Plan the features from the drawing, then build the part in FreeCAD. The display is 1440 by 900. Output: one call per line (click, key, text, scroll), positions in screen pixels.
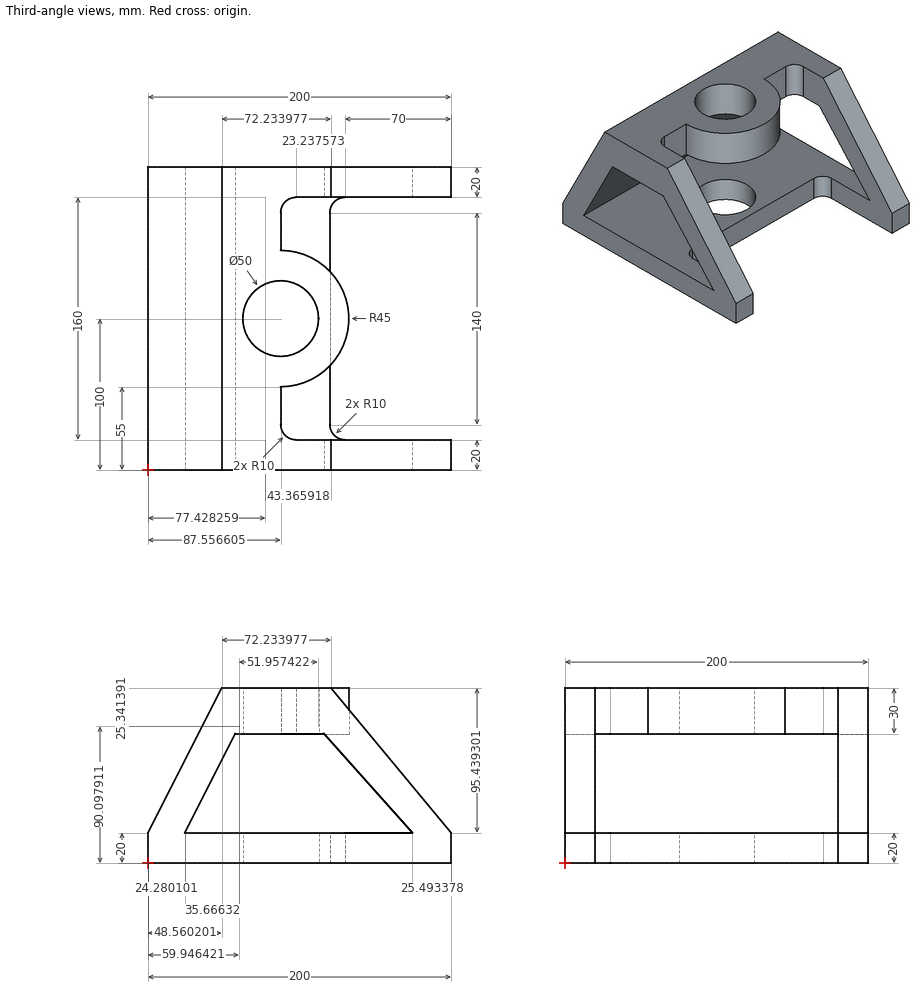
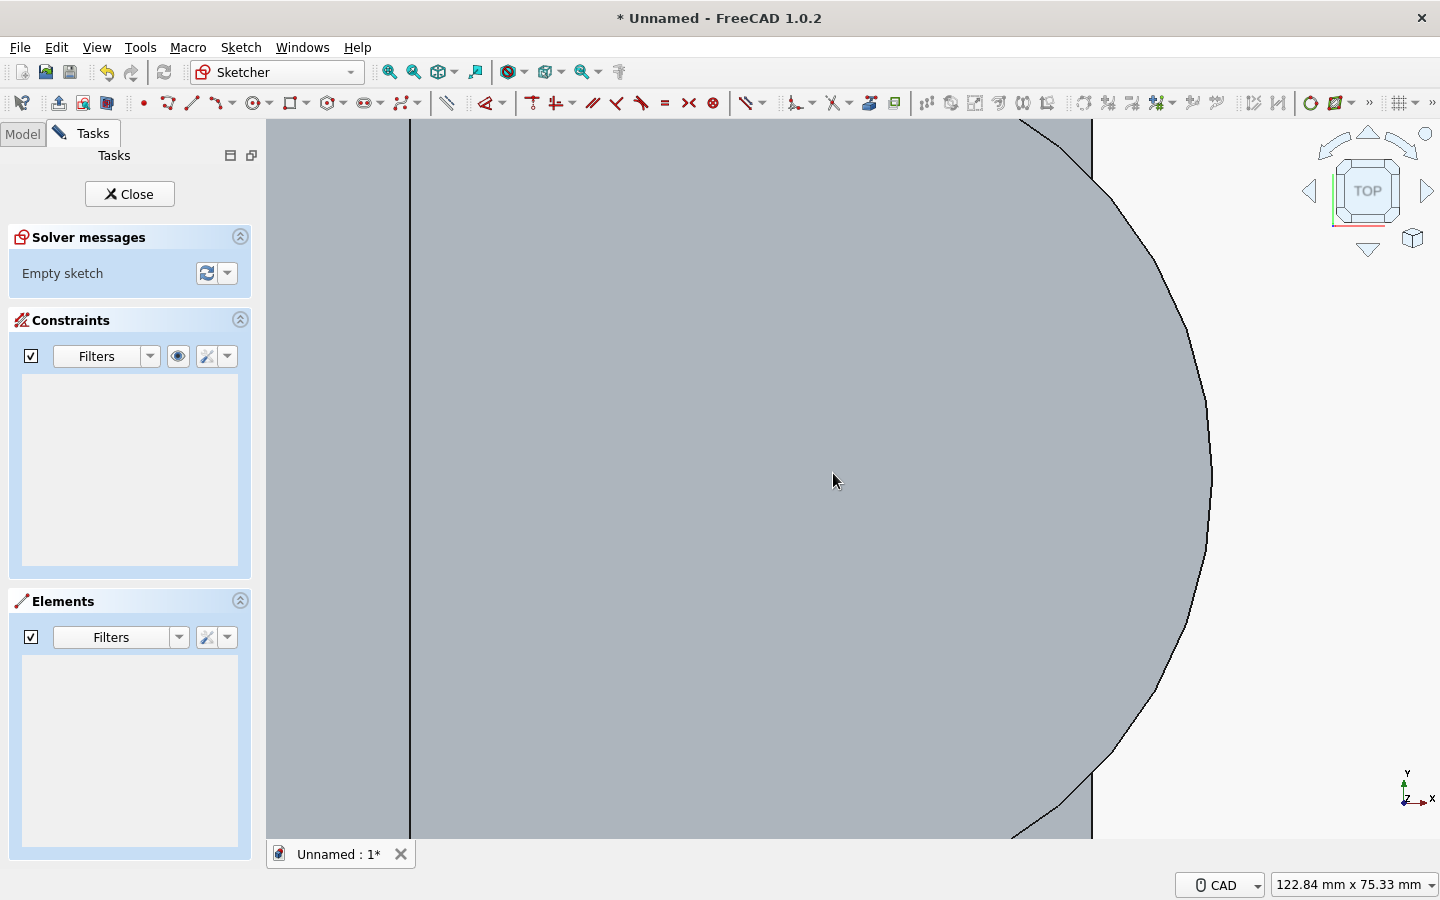
click(254, 104)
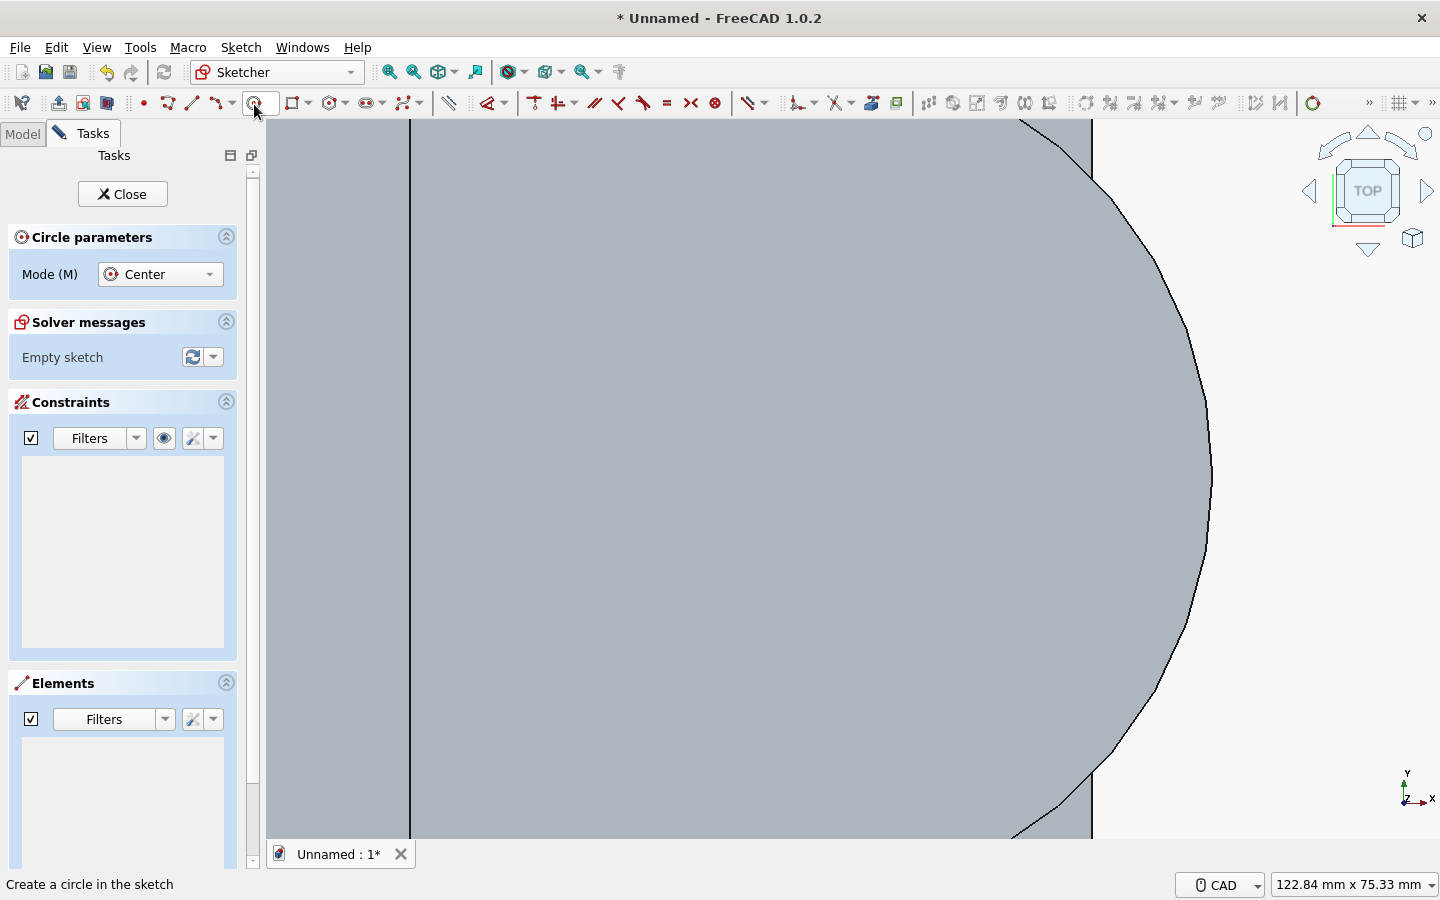
click(782, 476)
click(951, 307)
key(Escape)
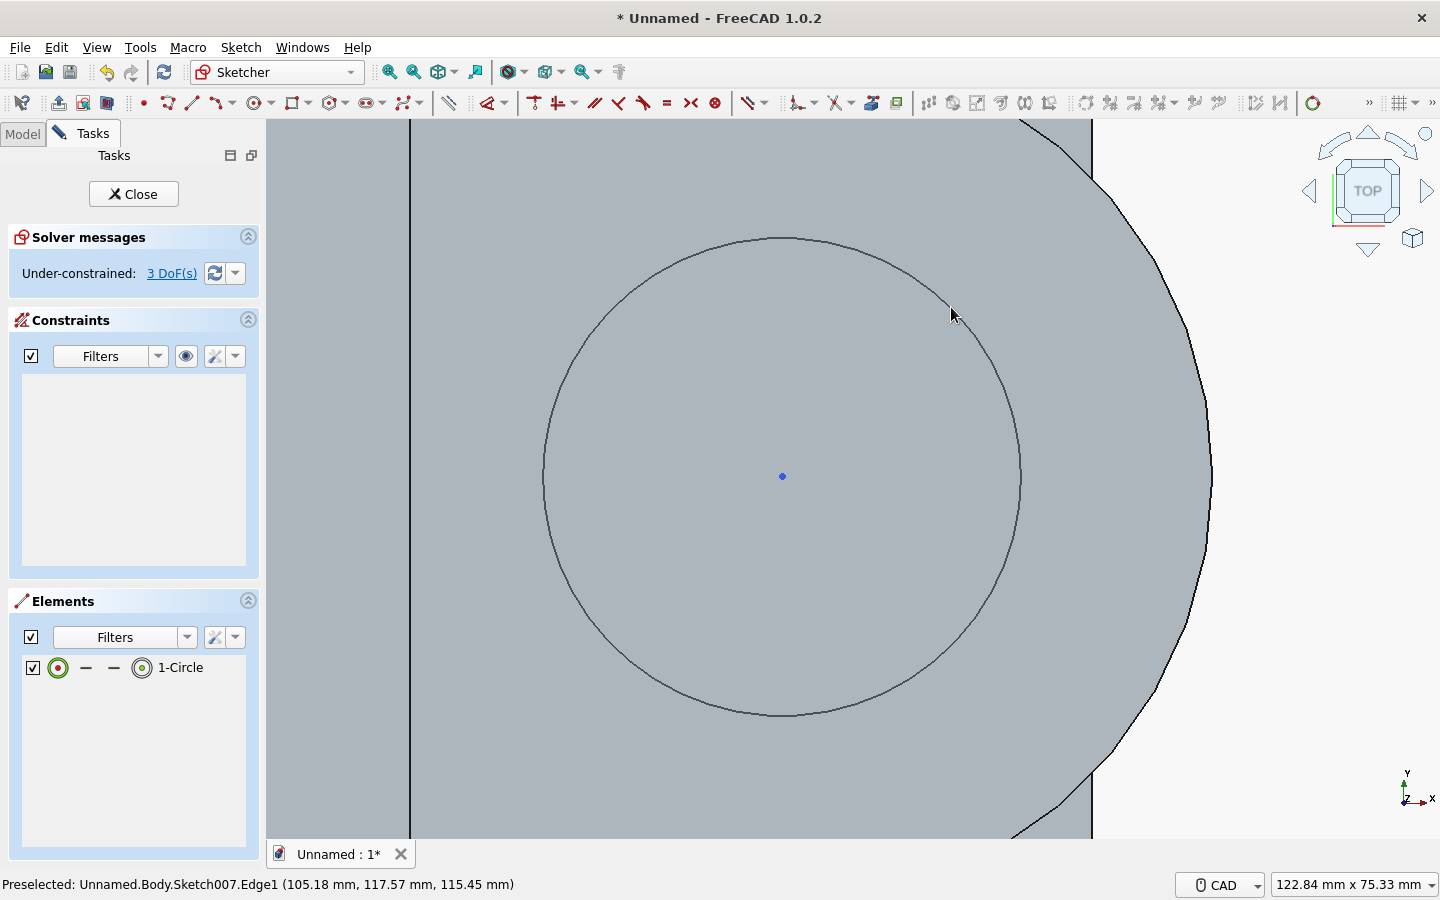
click(488, 104)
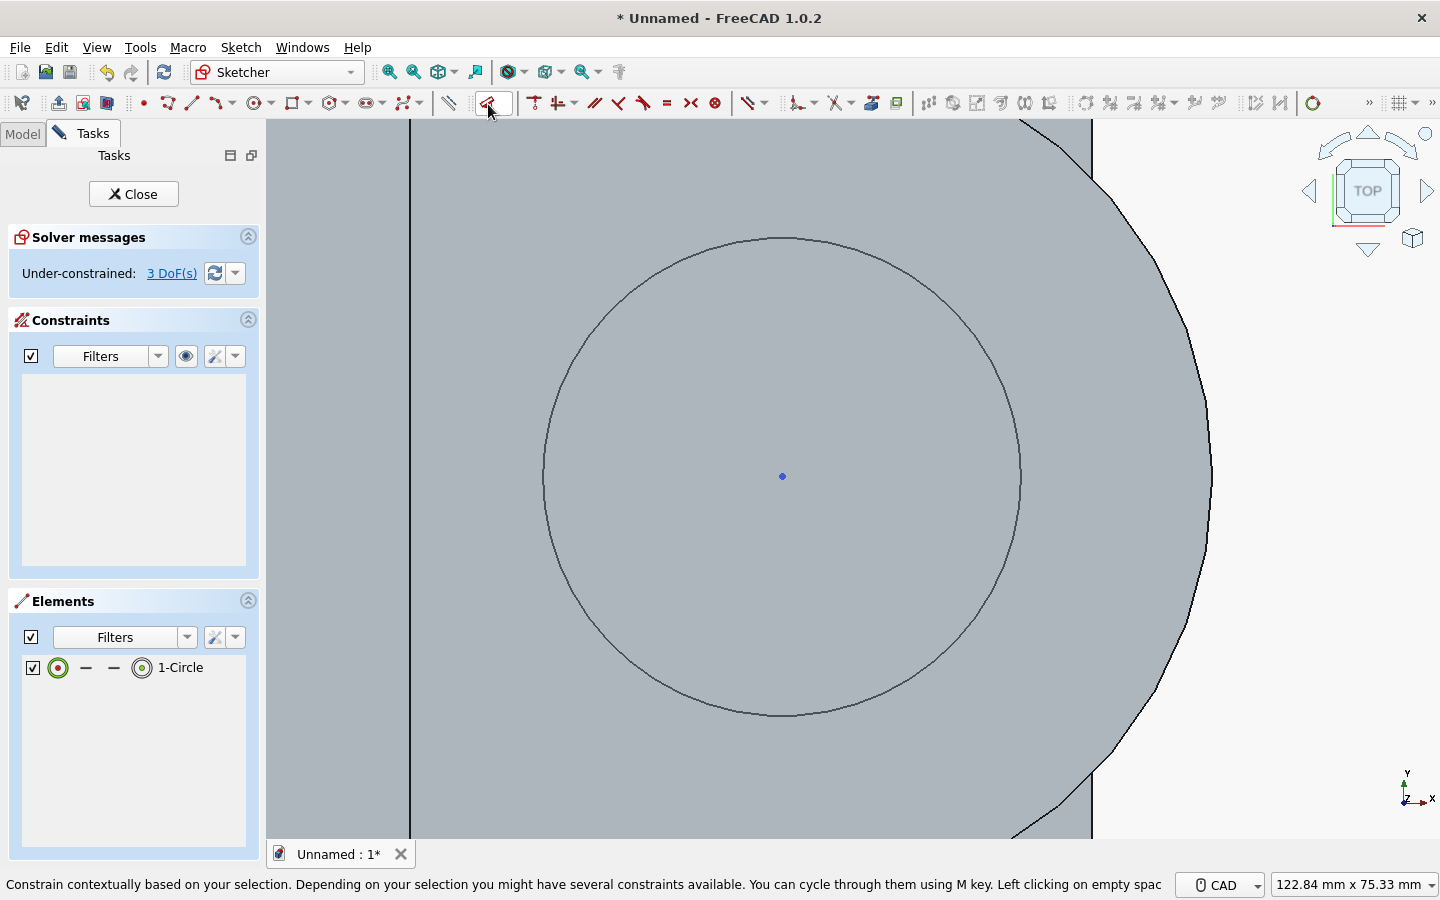
click(950, 307)
click(972, 284)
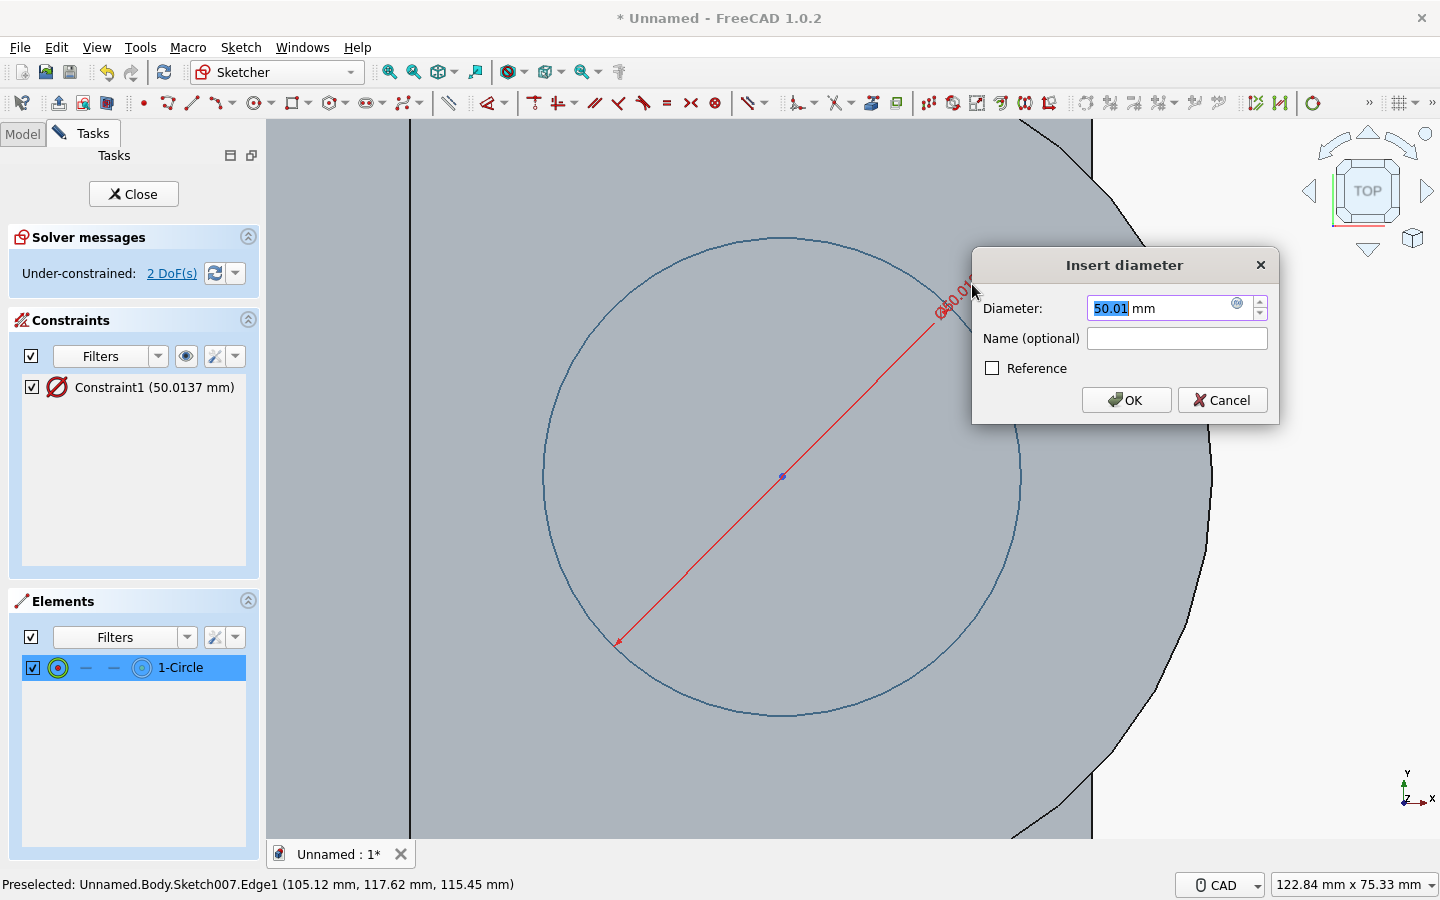
text(50)
key(Return)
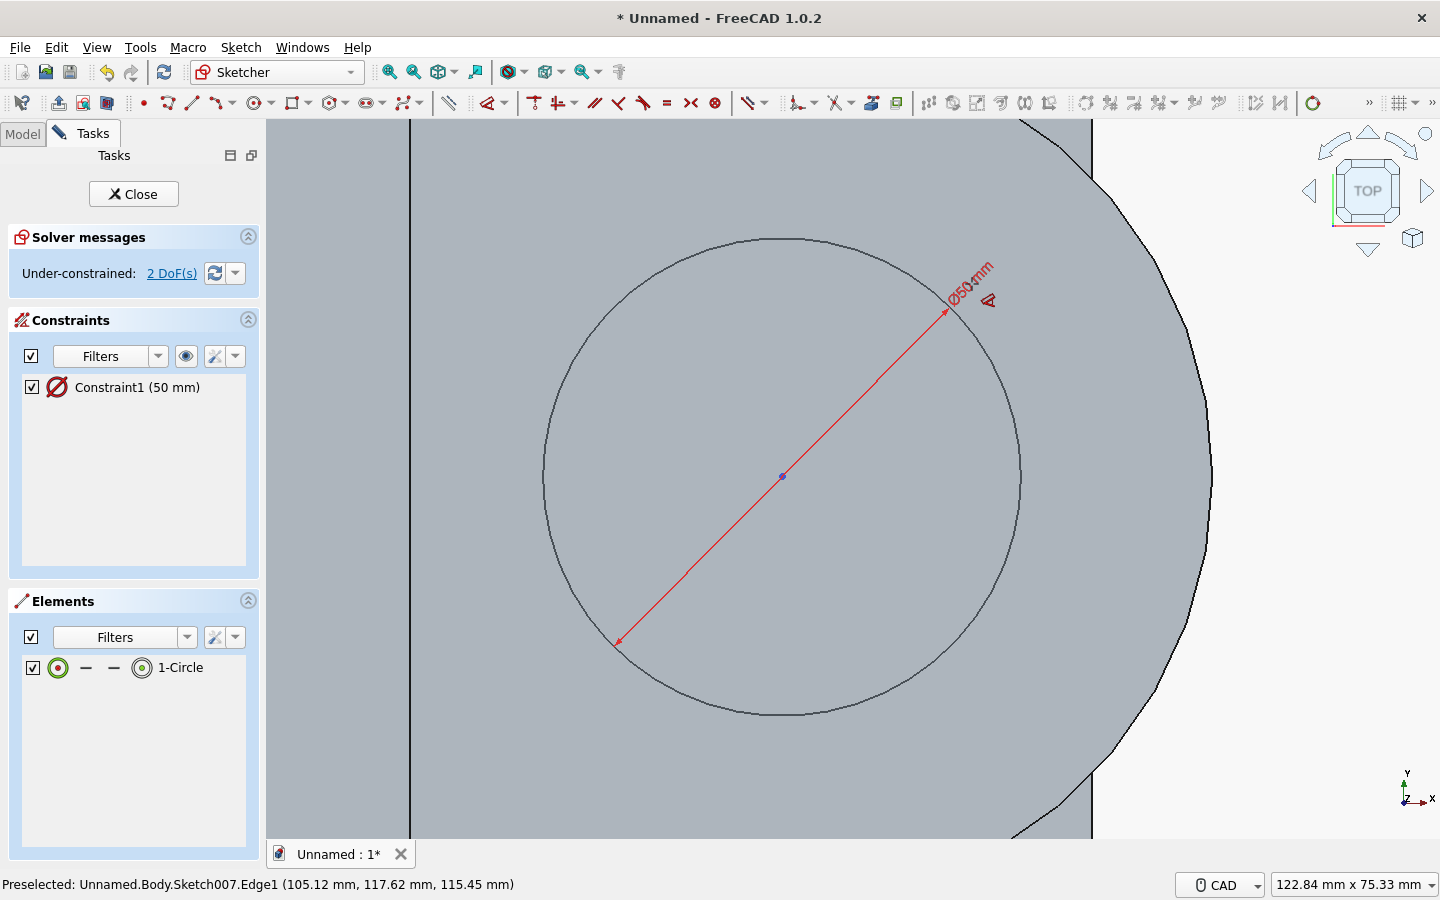
click(782, 477)
click(816, 644)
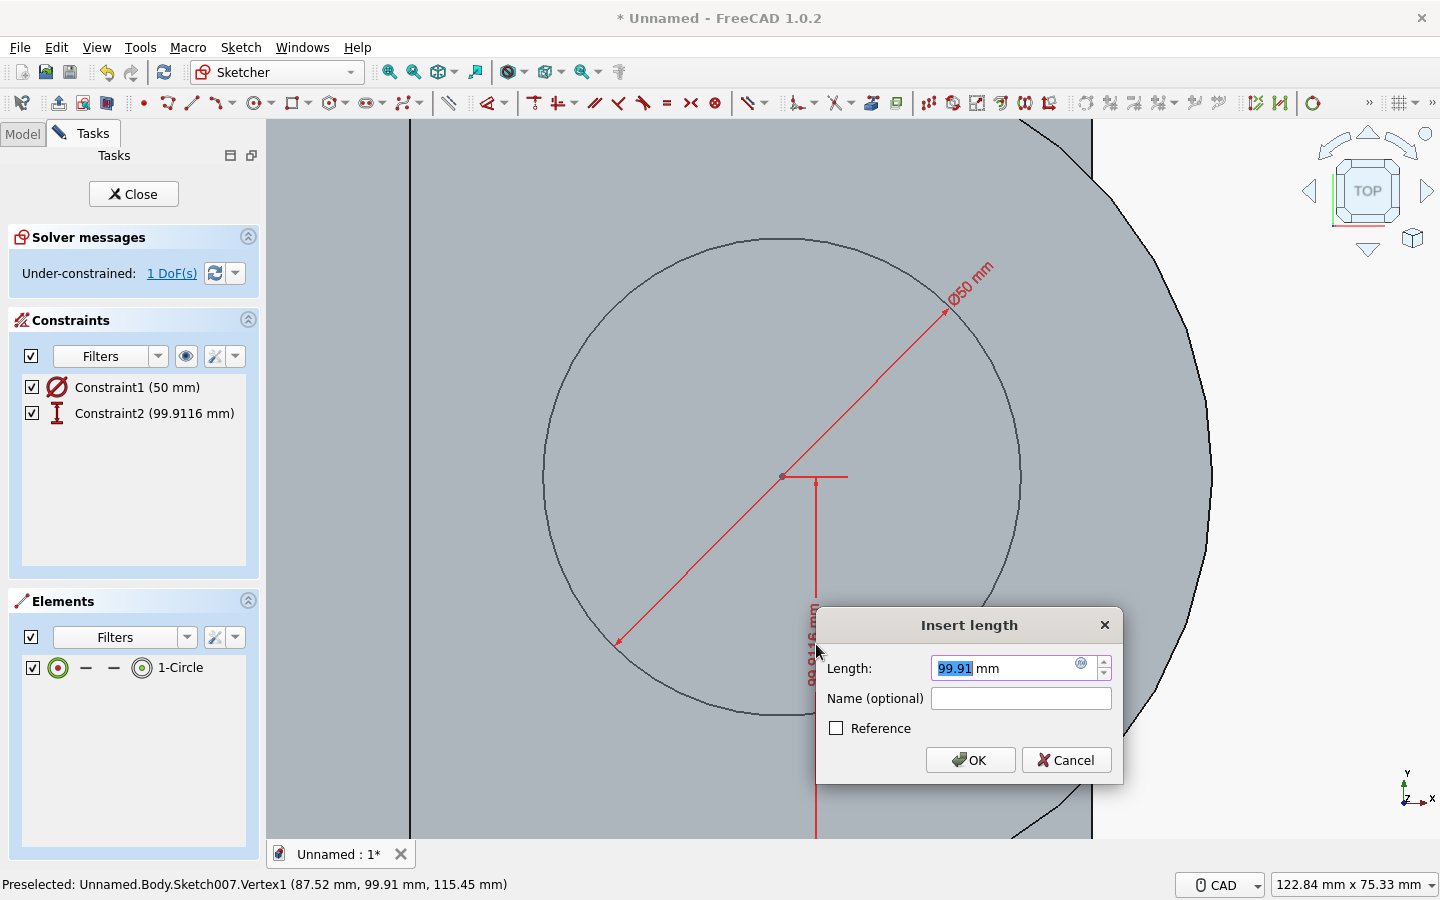
text(100)
key(Return)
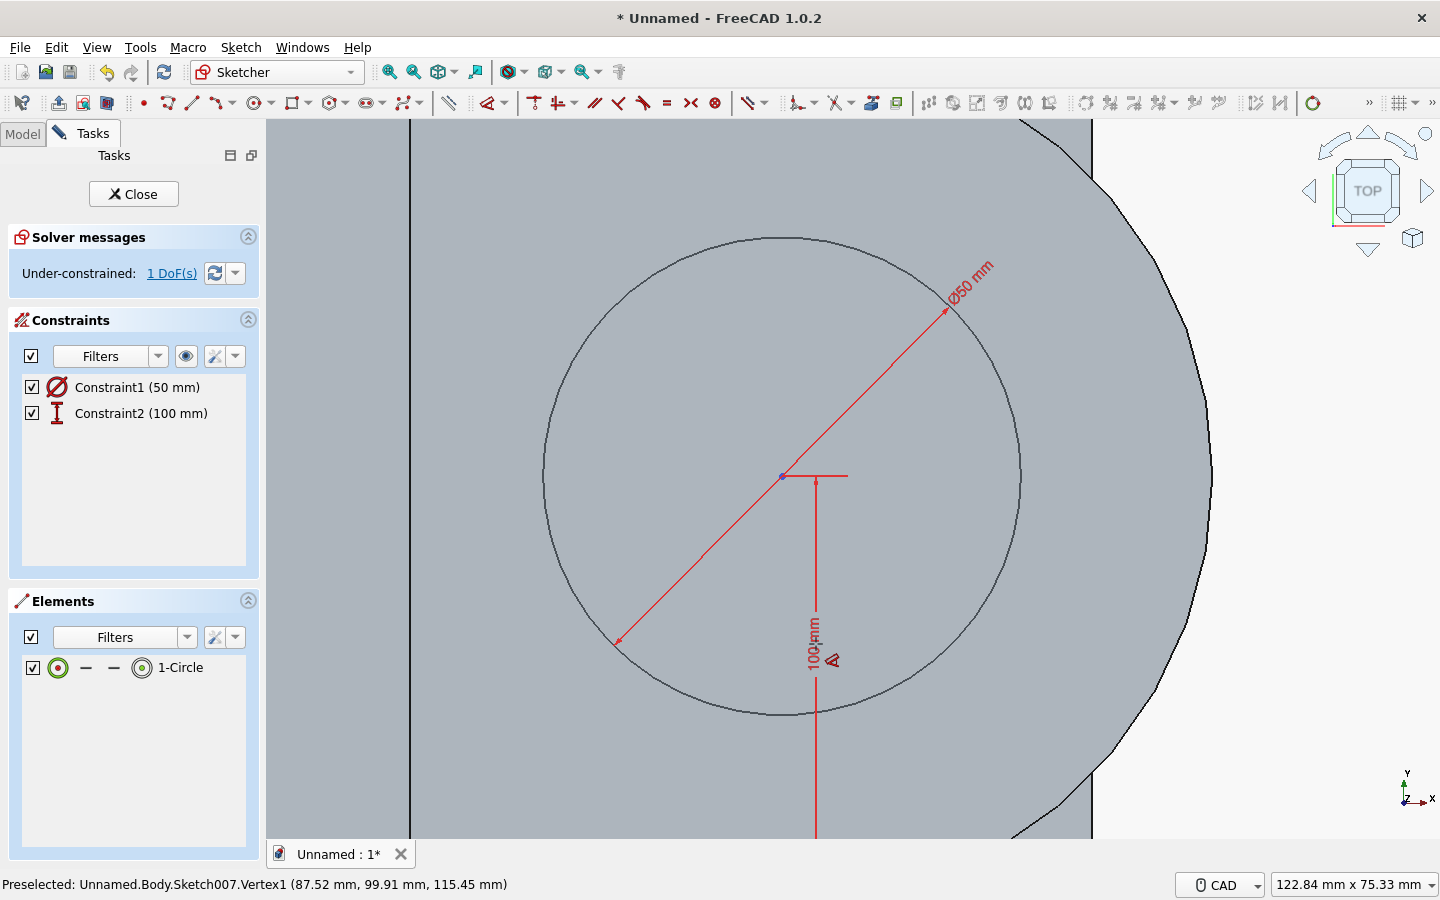
click(782, 476)
click(426, 442)